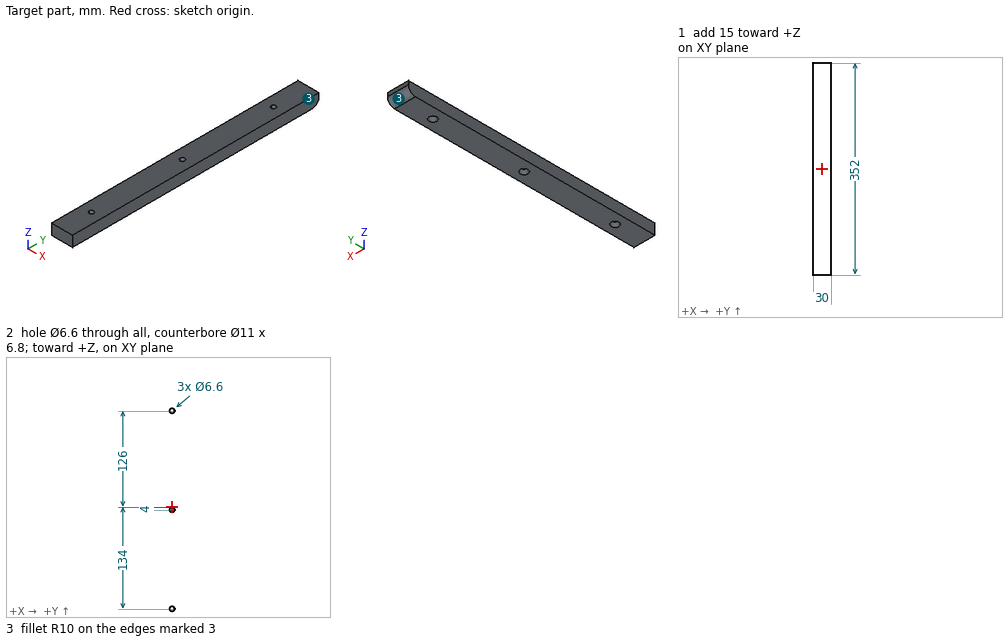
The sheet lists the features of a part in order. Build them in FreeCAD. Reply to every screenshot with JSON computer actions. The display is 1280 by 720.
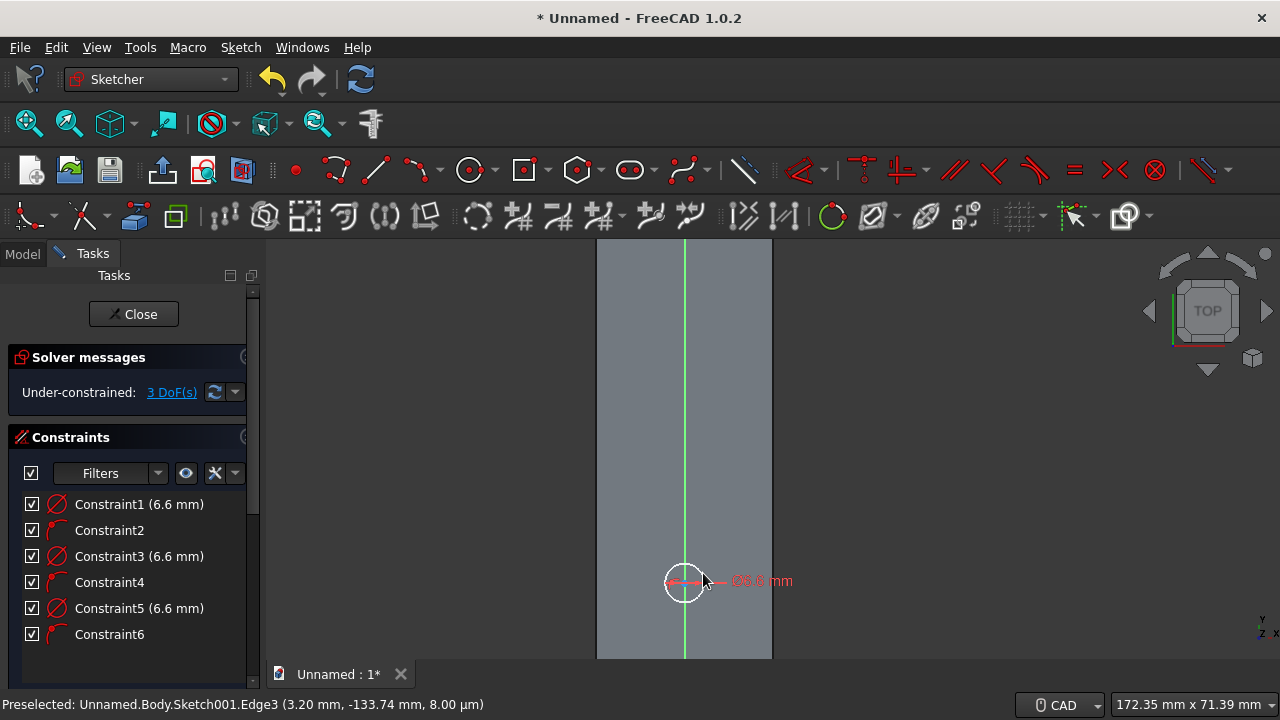
{"action": "left_click", "coordinate": [800, 170]}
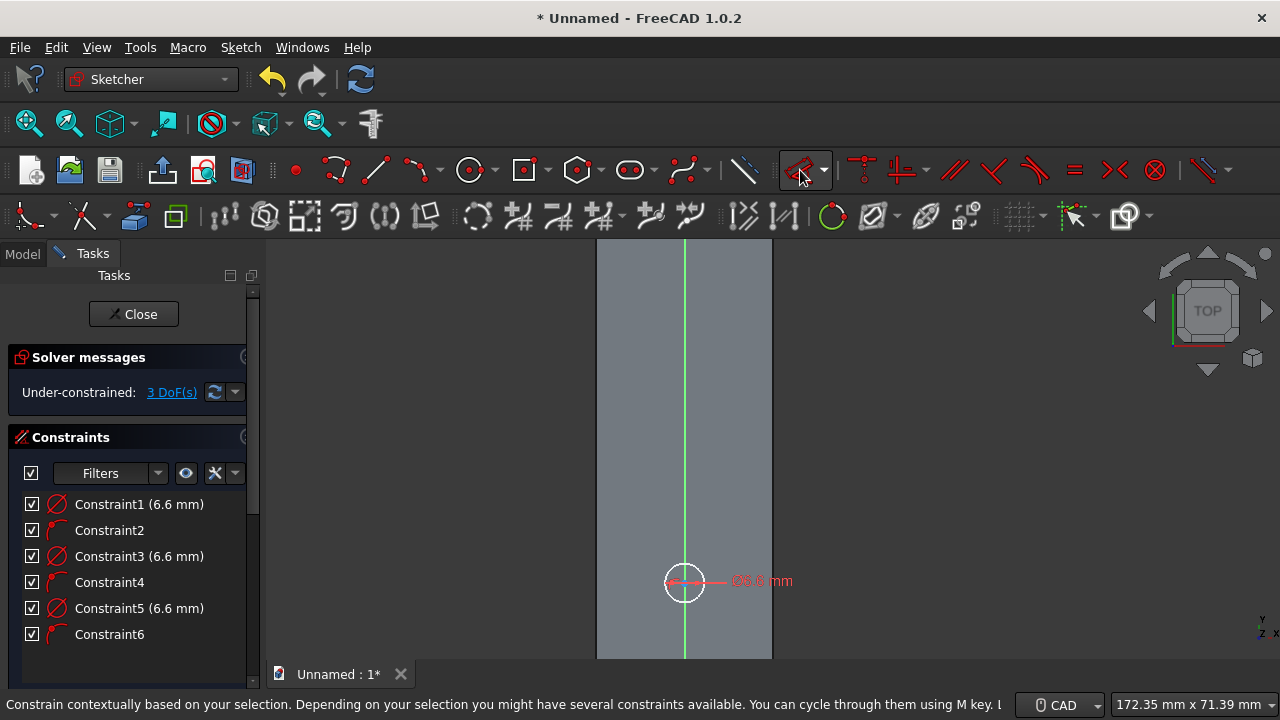
{"action": "scroll", "coordinate": [708, 575], "scroll_direction": "down", "scroll_amount": 9}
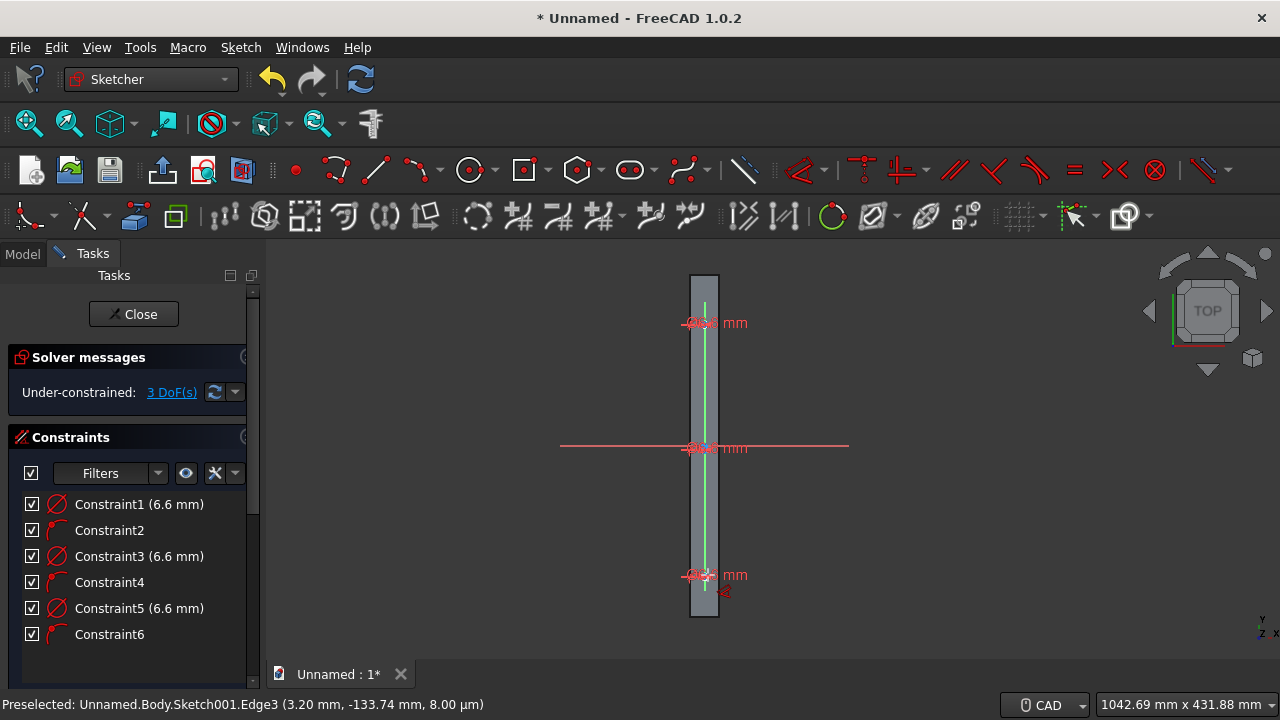
{"action": "scroll", "coordinate": [705, 450], "scroll_direction": "up", "scroll_amount": 12}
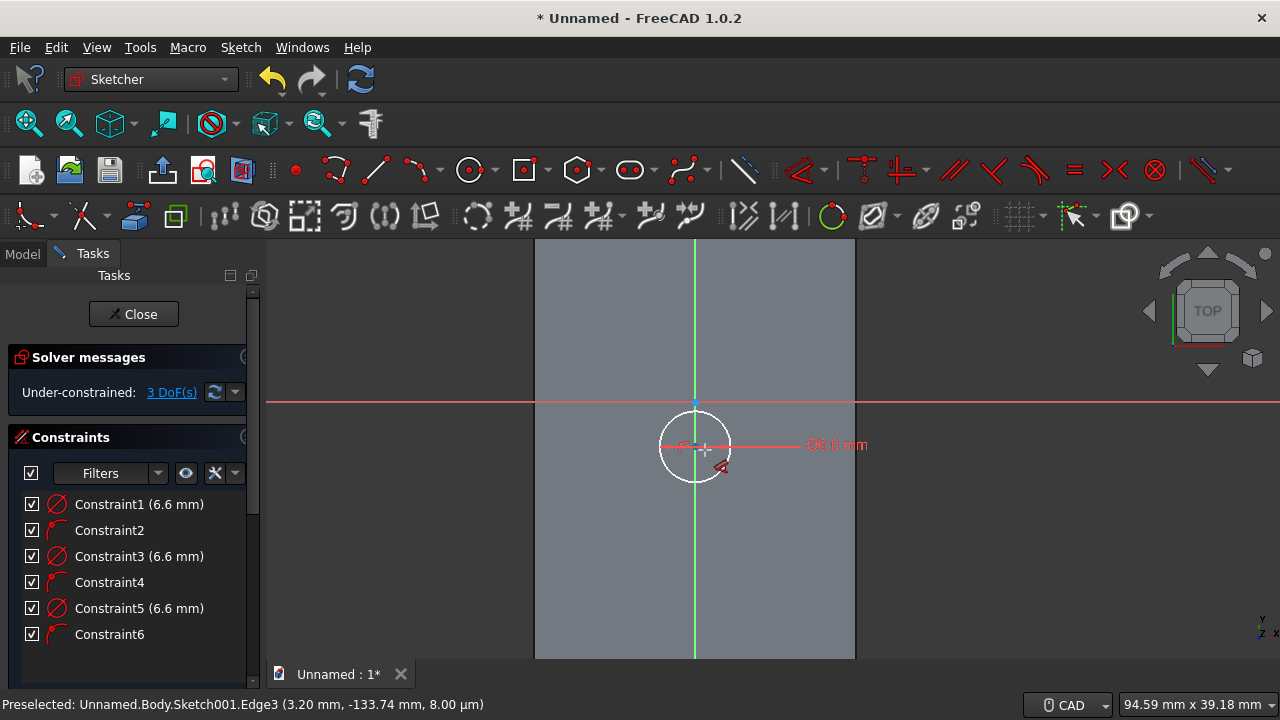
{"action": "left_click", "coordinate": [695, 447]}
{"action": "left_click", "coordinate": [753, 425]}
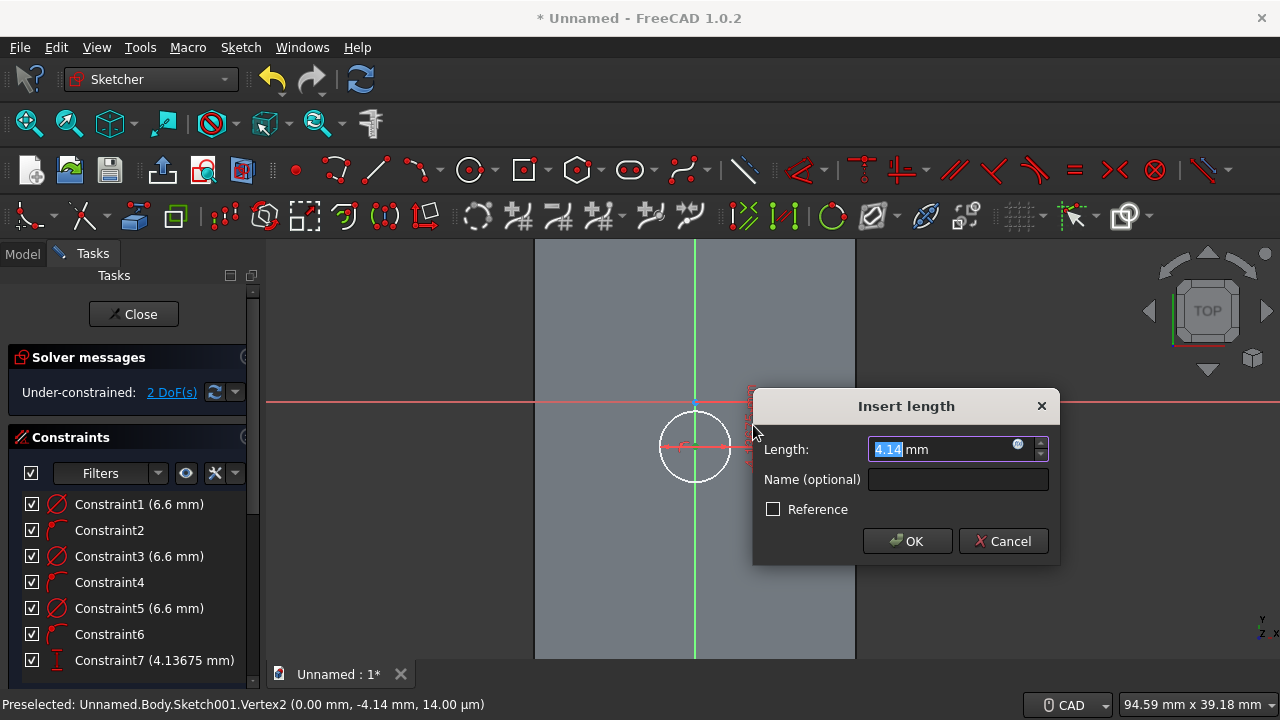
{"action": "type", "text": "4"}
{"action": "key", "text": "Return"}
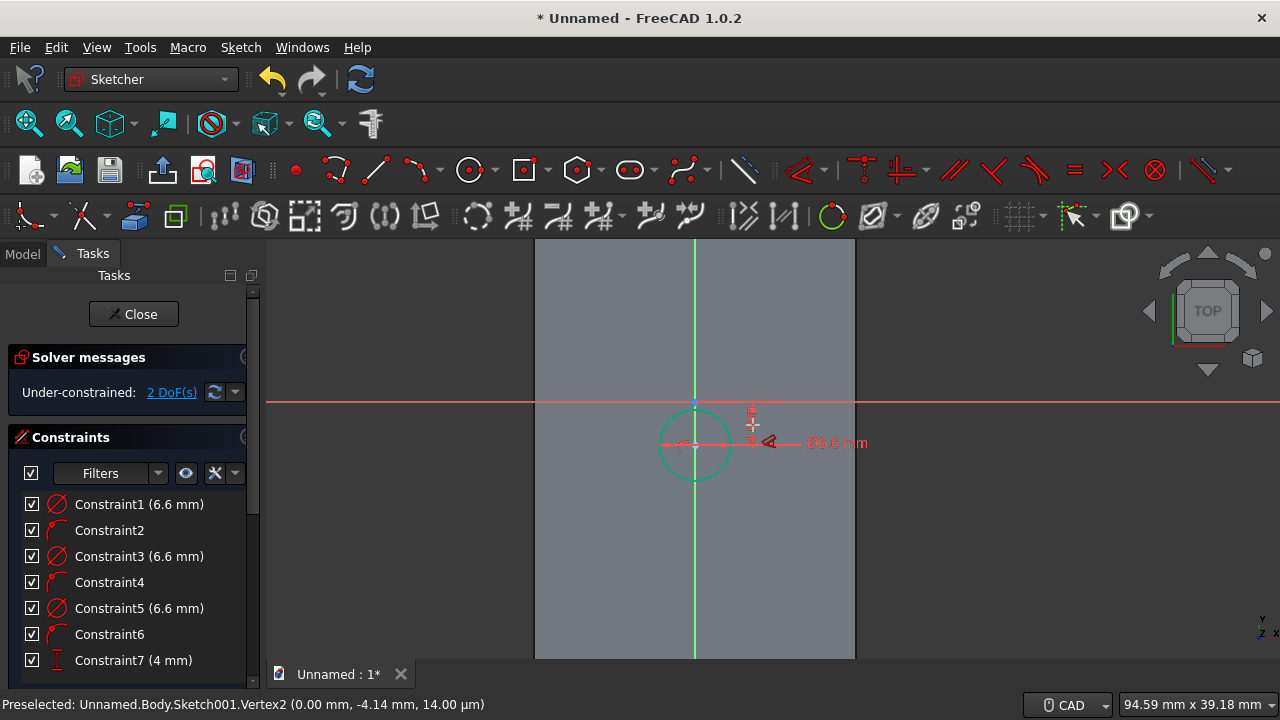
{"action": "scroll", "coordinate": [705, 449], "scroll_direction": "down", "scroll_amount": 12}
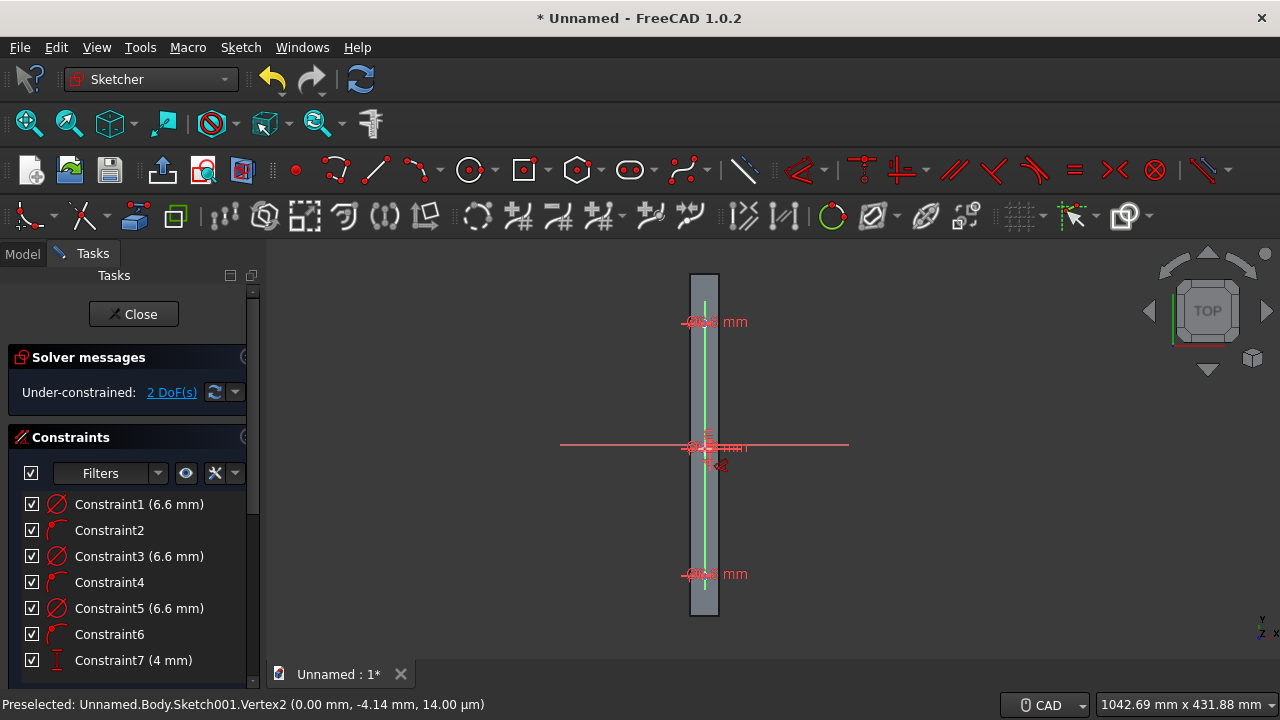
{"action": "left_click", "coordinate": [705, 324]}
{"action": "left_click", "coordinate": [739, 385]}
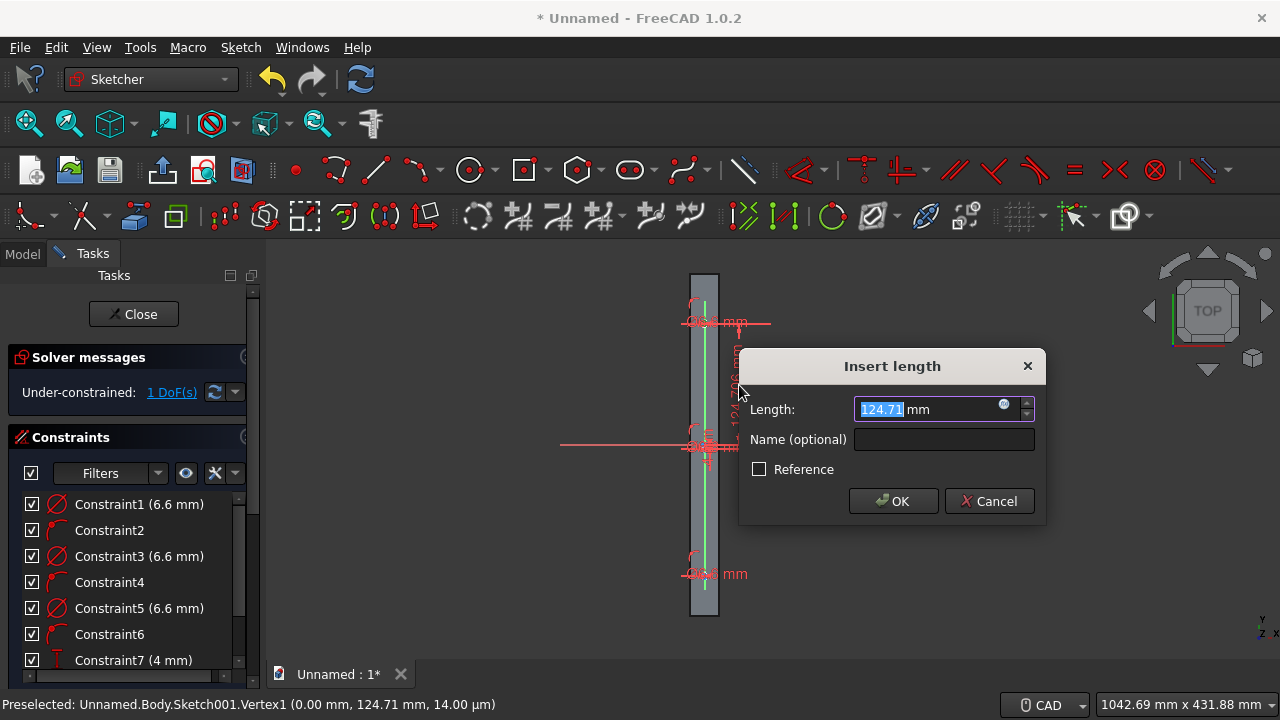
{"action": "type", "text": "126"}
{"action": "key", "text": "Return"}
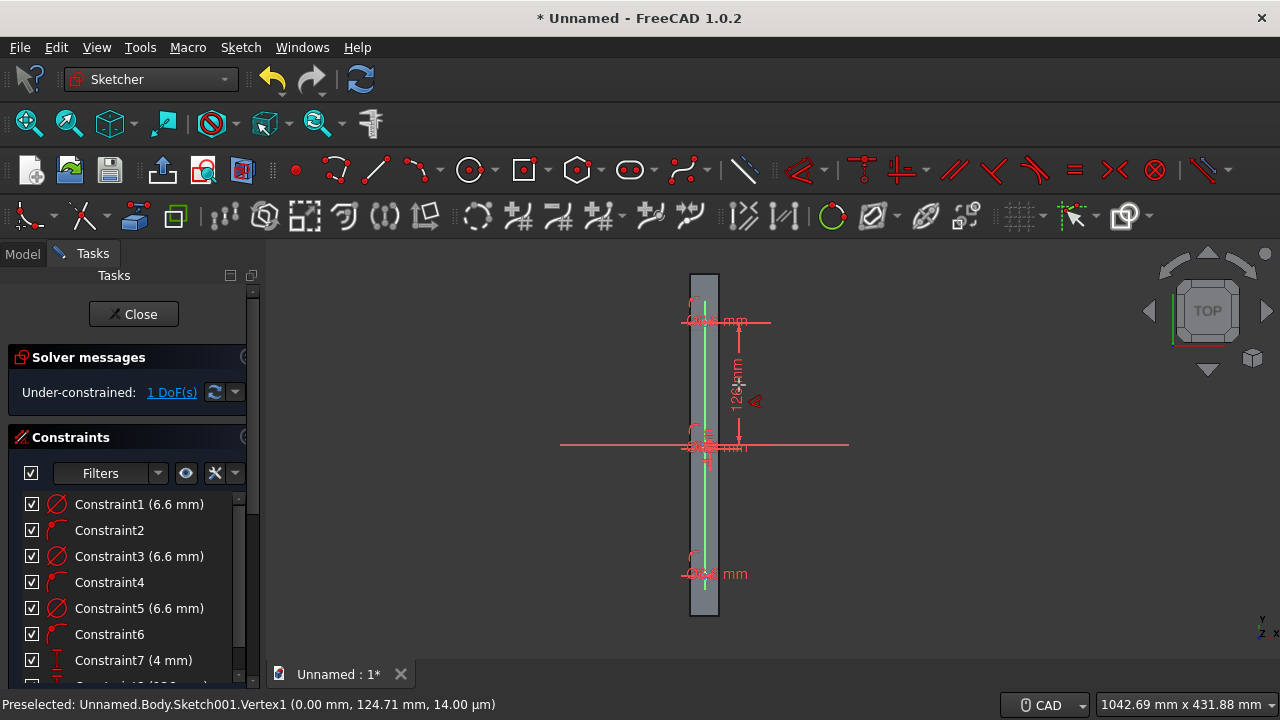
{"action": "left_click", "coordinate": [705, 576]}
{"action": "left_click", "coordinate": [739, 511]}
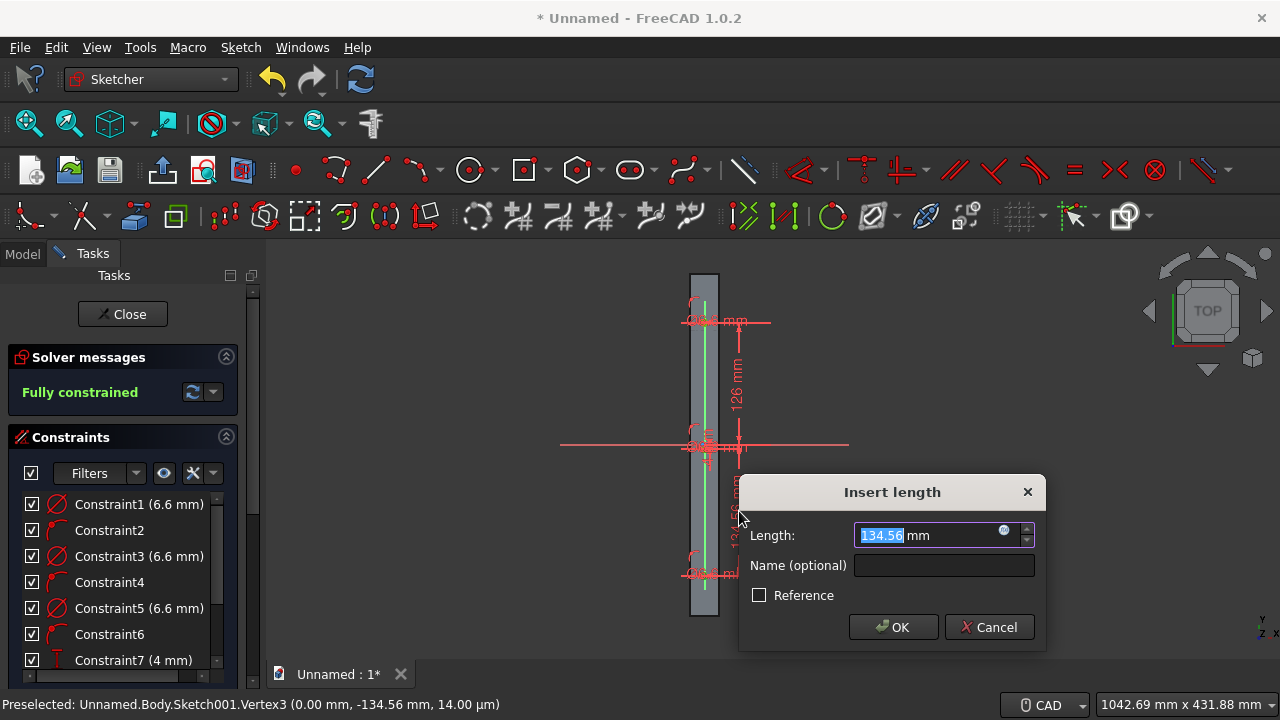
{"action": "type", "text": "134"}
{"action": "key", "text": "Return"}
{"action": "key", "text": "Escape"}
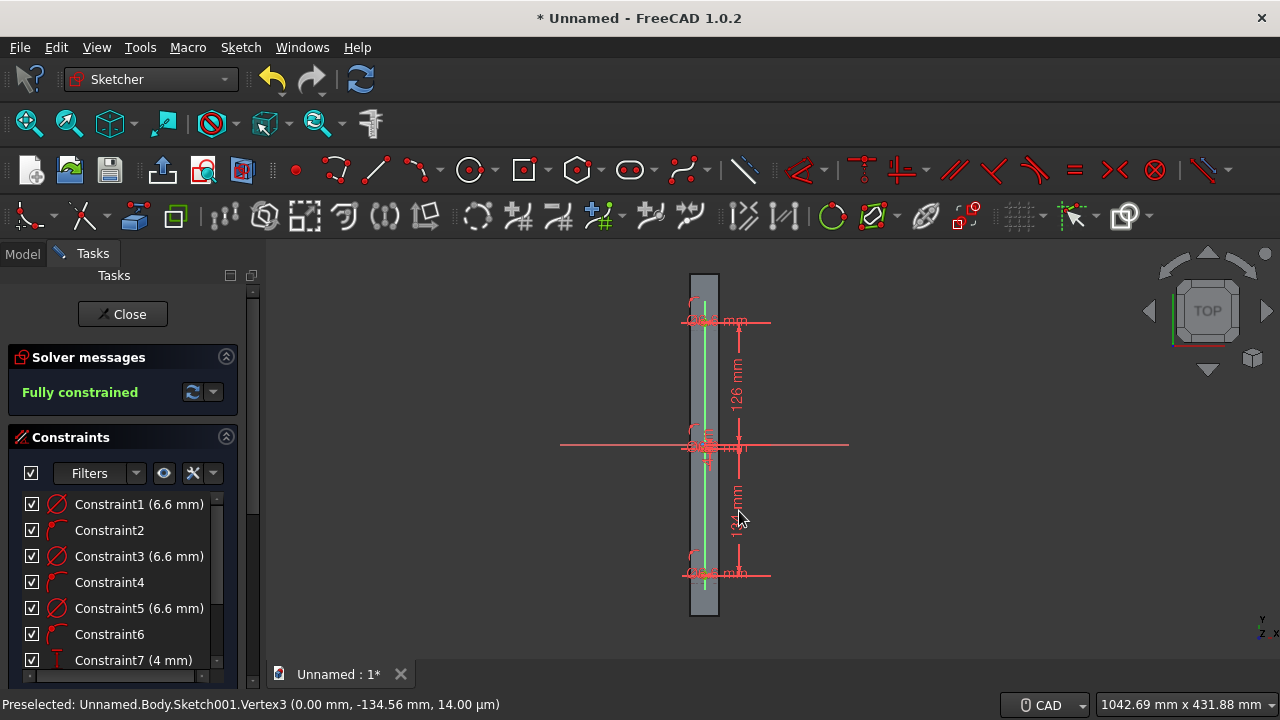
{"action": "left_click", "coordinate": [123, 314]}